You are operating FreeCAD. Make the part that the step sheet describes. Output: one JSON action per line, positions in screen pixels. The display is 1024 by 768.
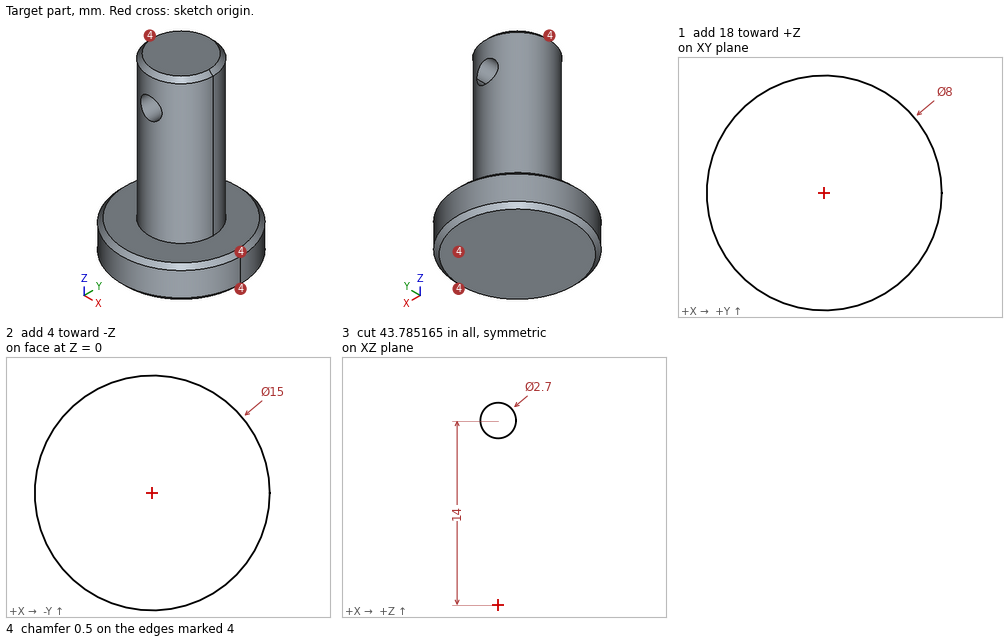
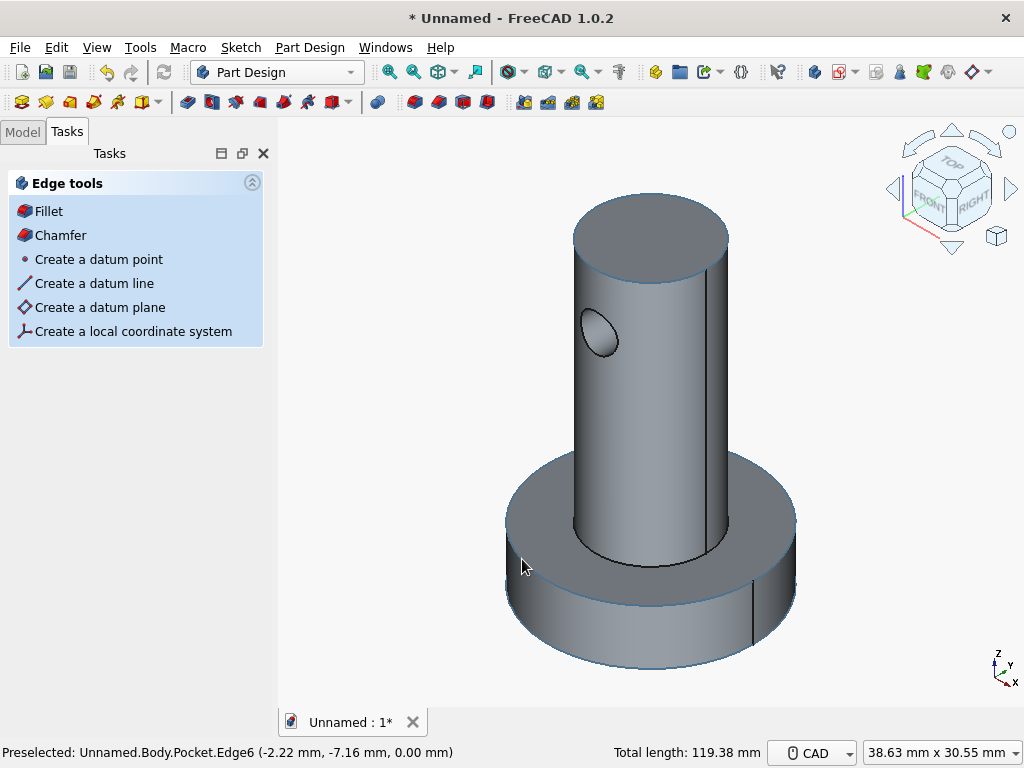
{"action": "left_click", "coordinate": [440, 102]}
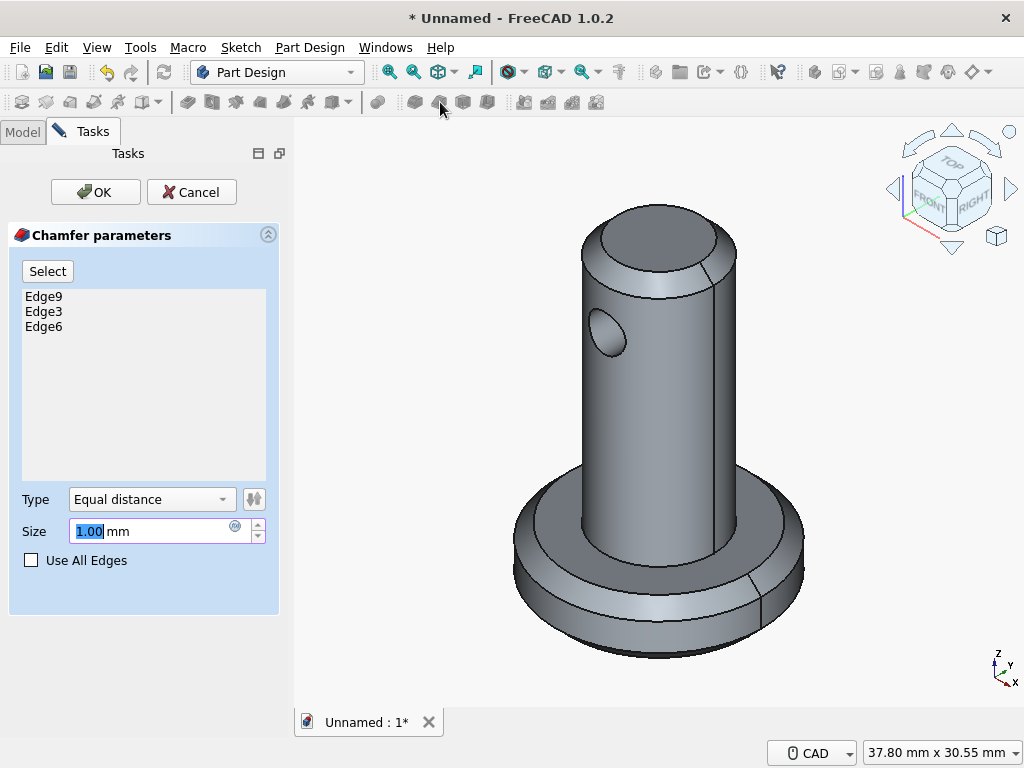
{"action": "type", "text": "0.5"}
{"action": "key", "text": "Tab"}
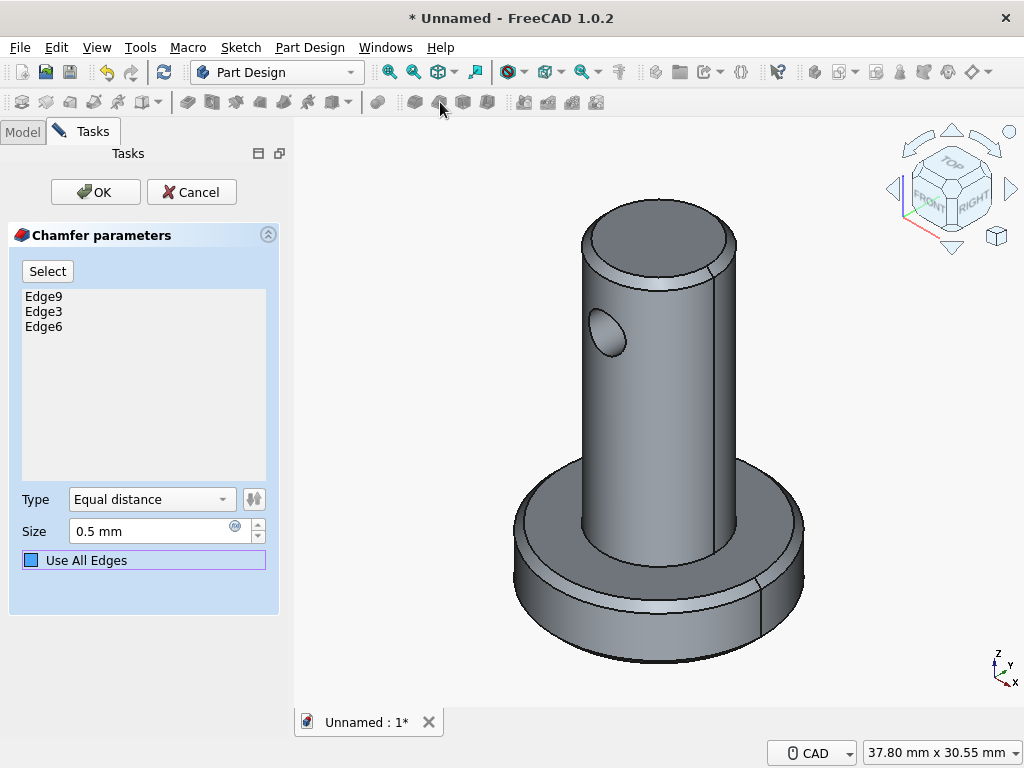
{"action": "left_click", "coordinate": [96, 192]}